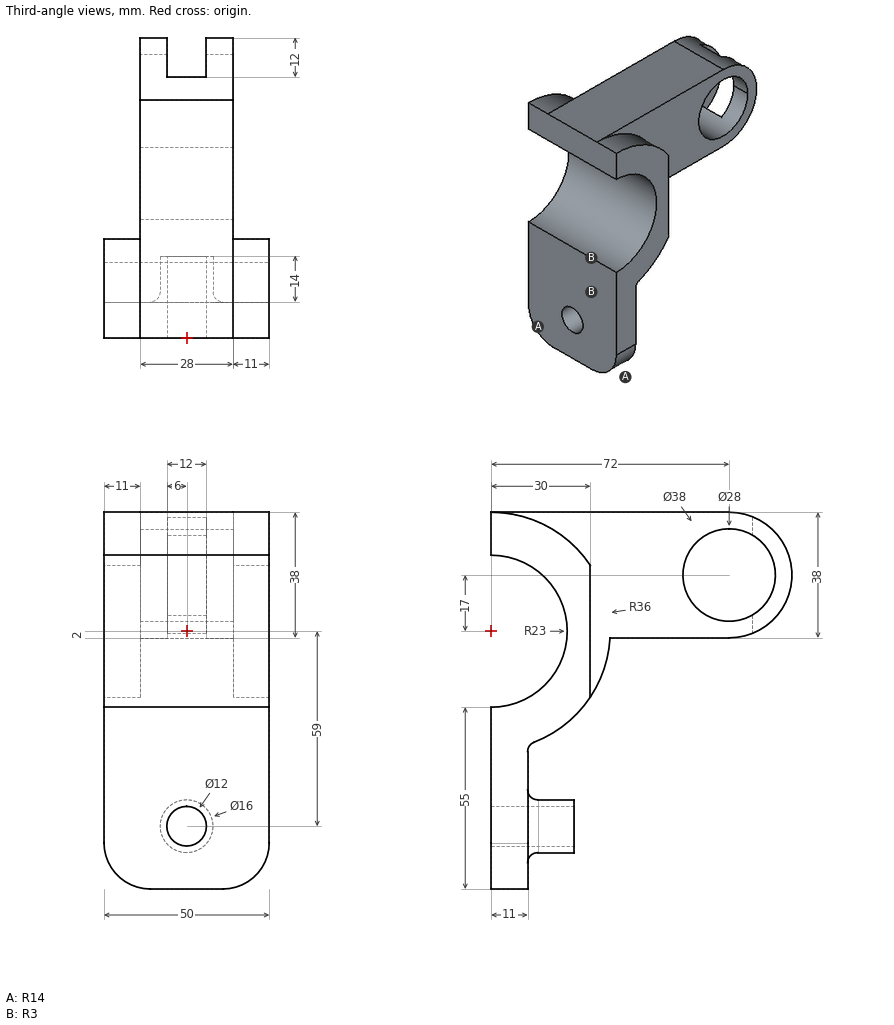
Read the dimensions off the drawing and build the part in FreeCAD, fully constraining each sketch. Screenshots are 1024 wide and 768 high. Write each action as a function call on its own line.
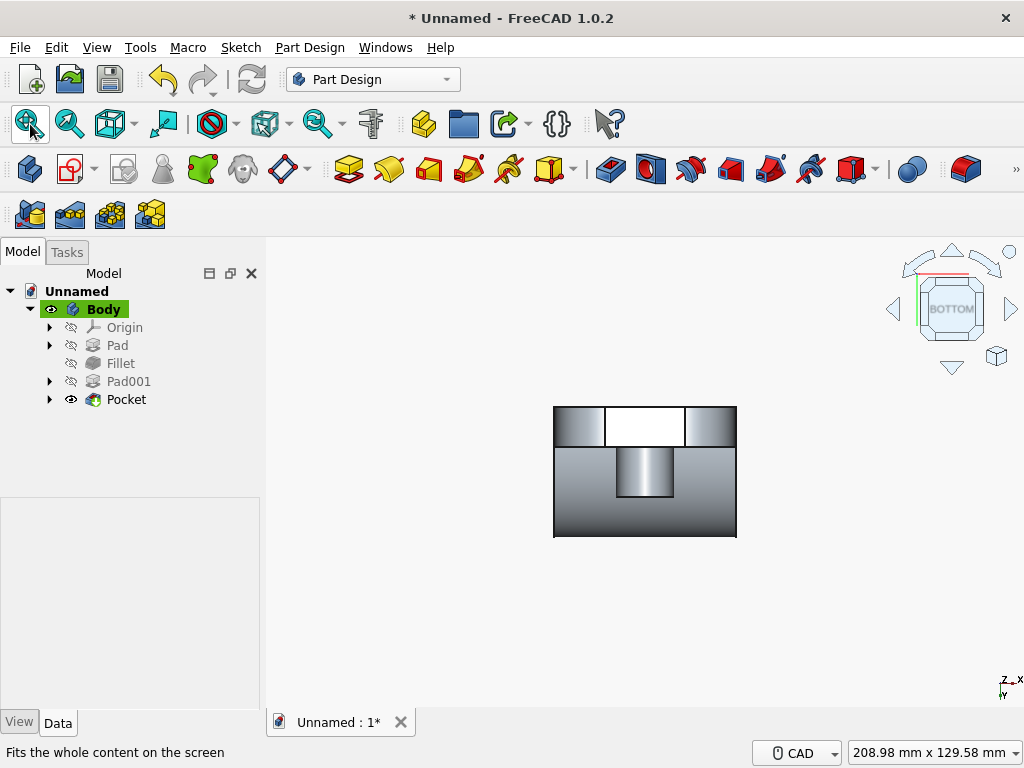
key(4)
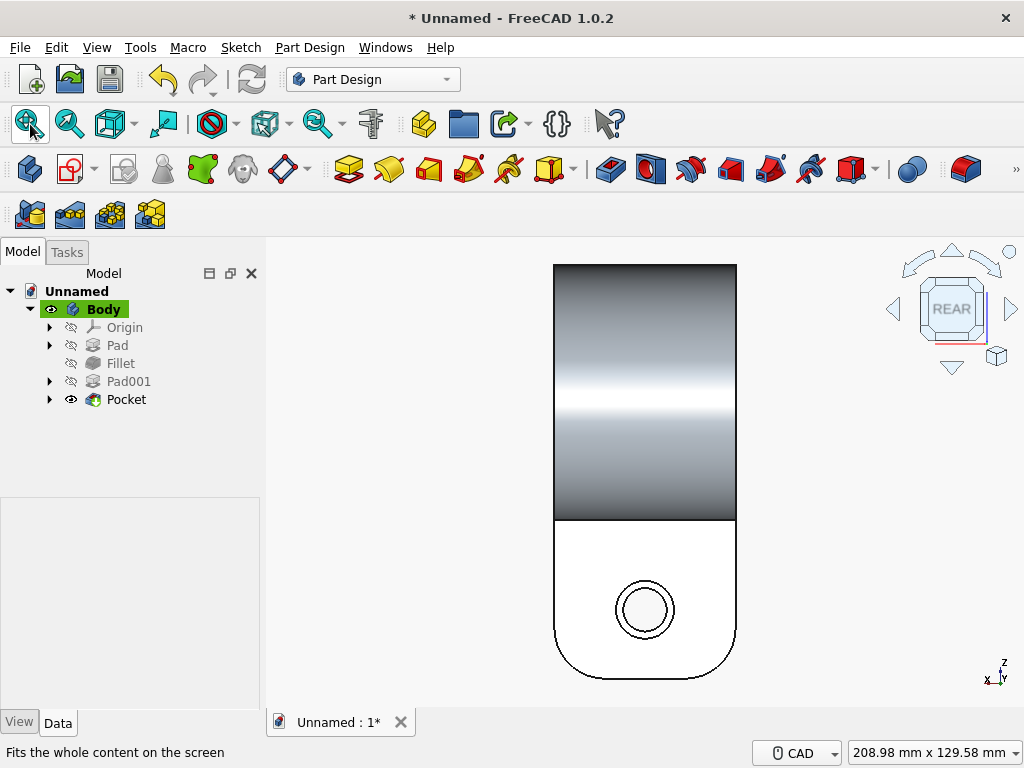
key(6)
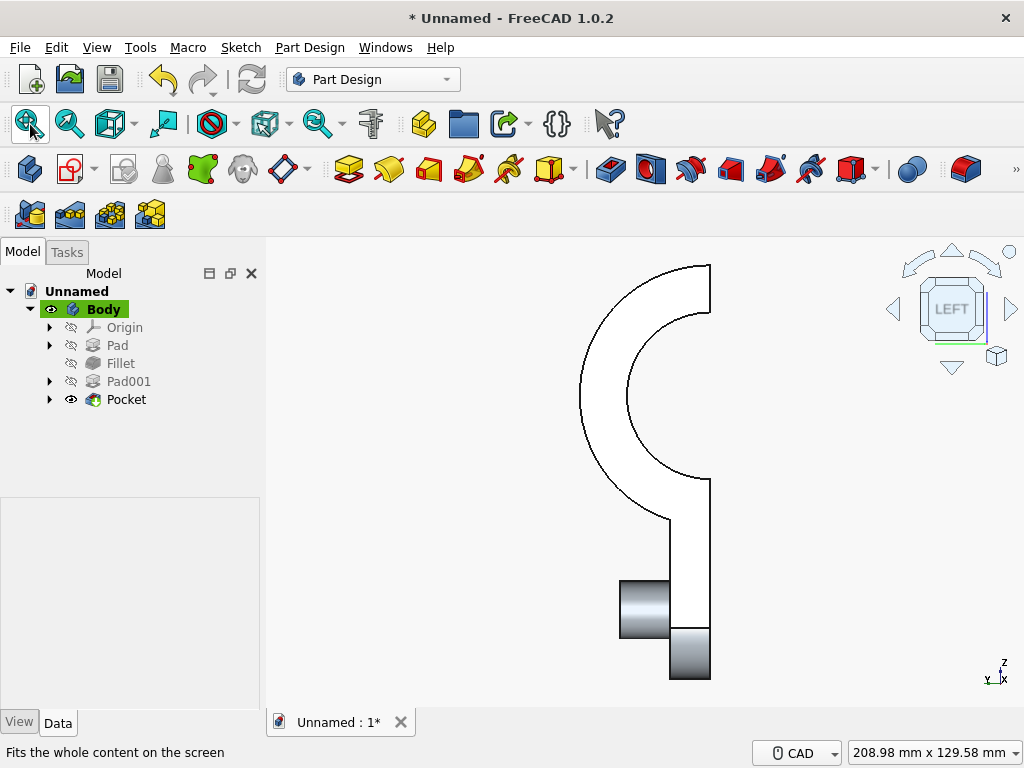
key(v)
key(3)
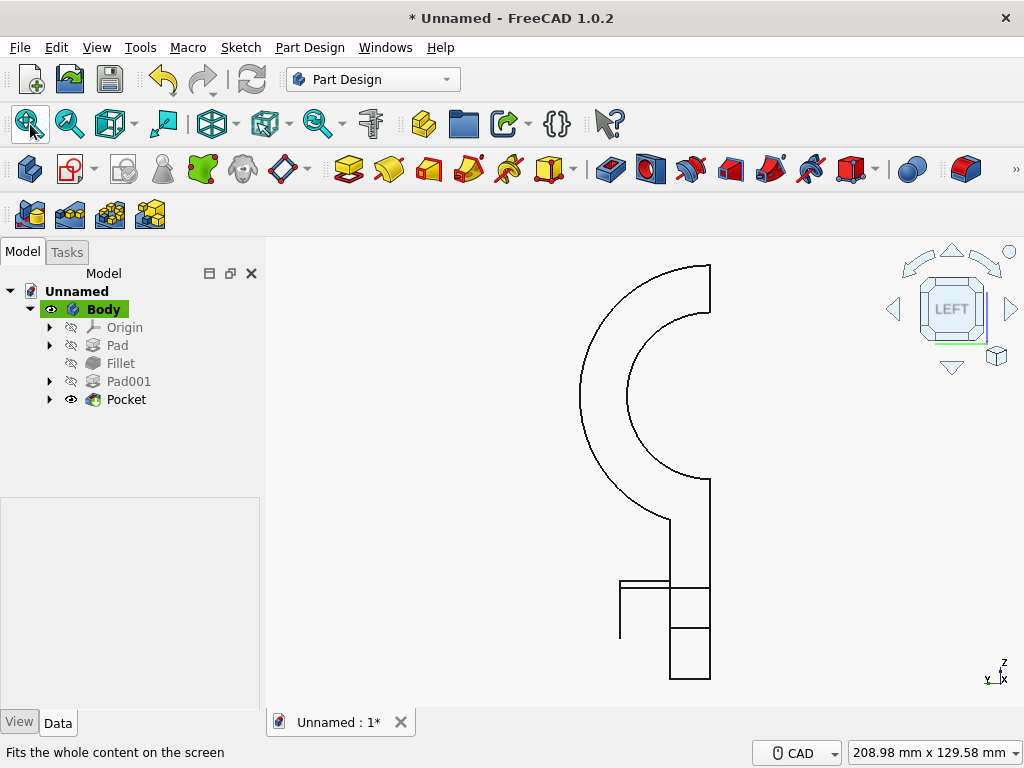
key(0)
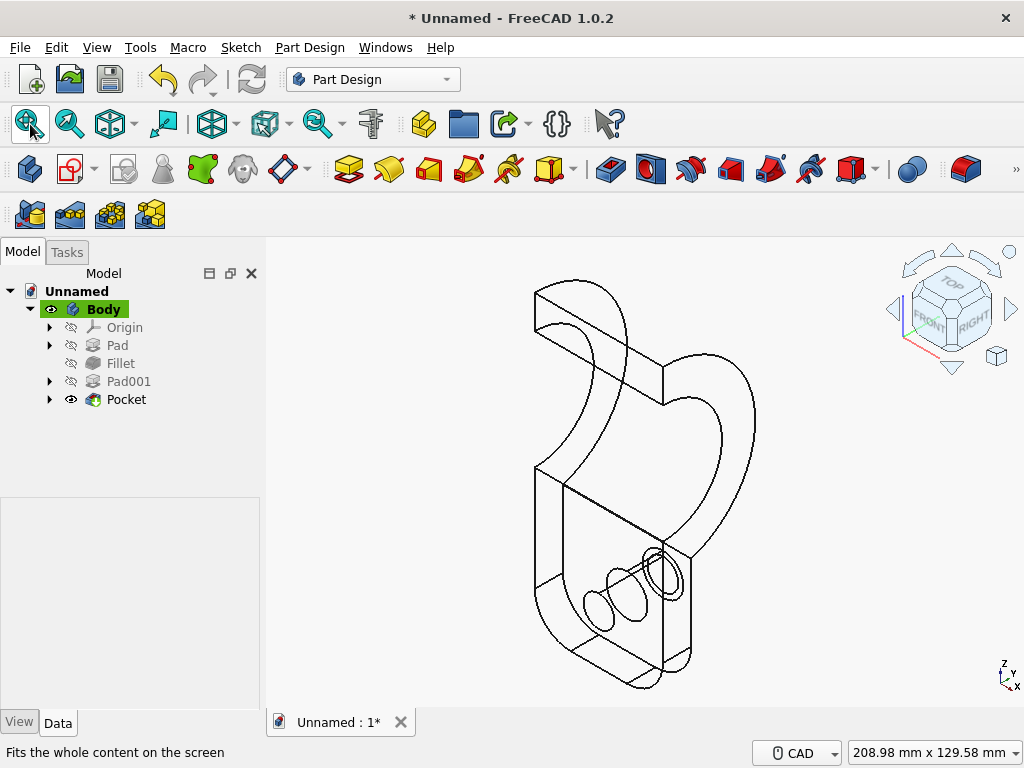
click(676, 549)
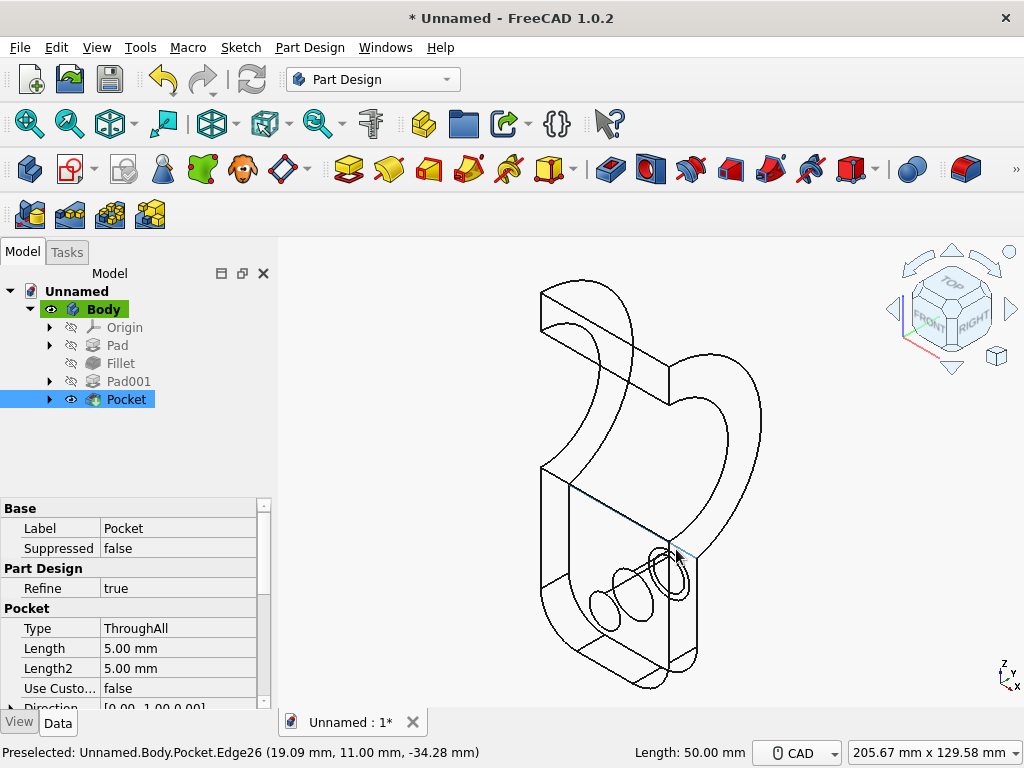
click(633, 618, ctrl)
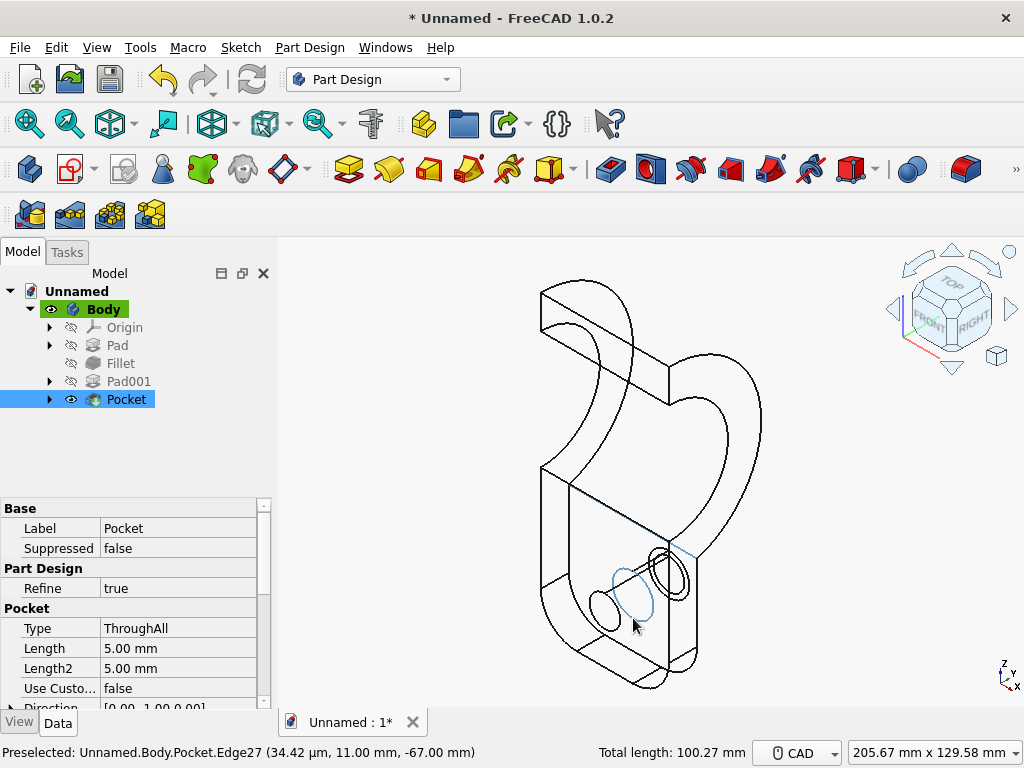
key(v)
key(1)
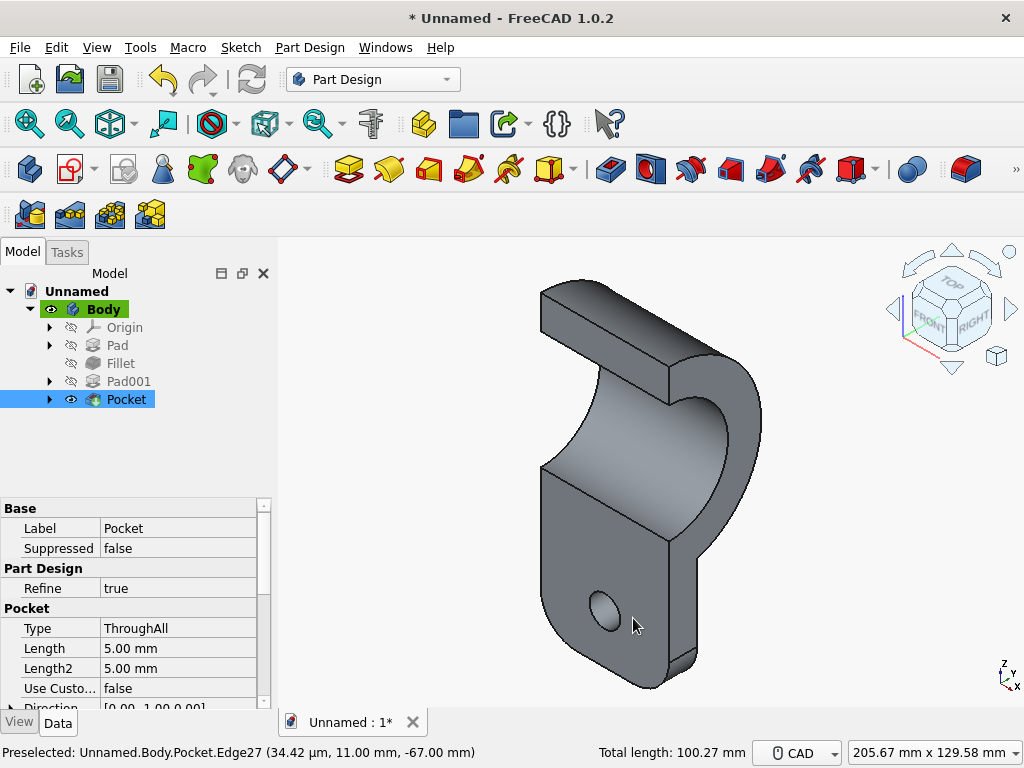
click(966, 170)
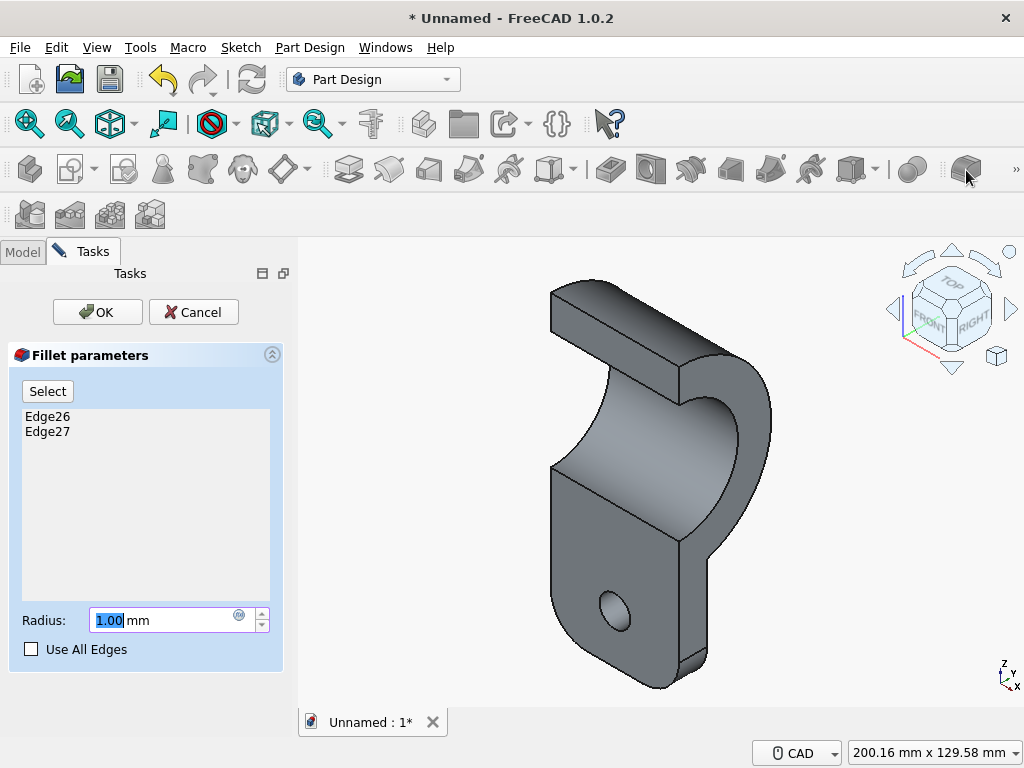
text(3)
key(Tab)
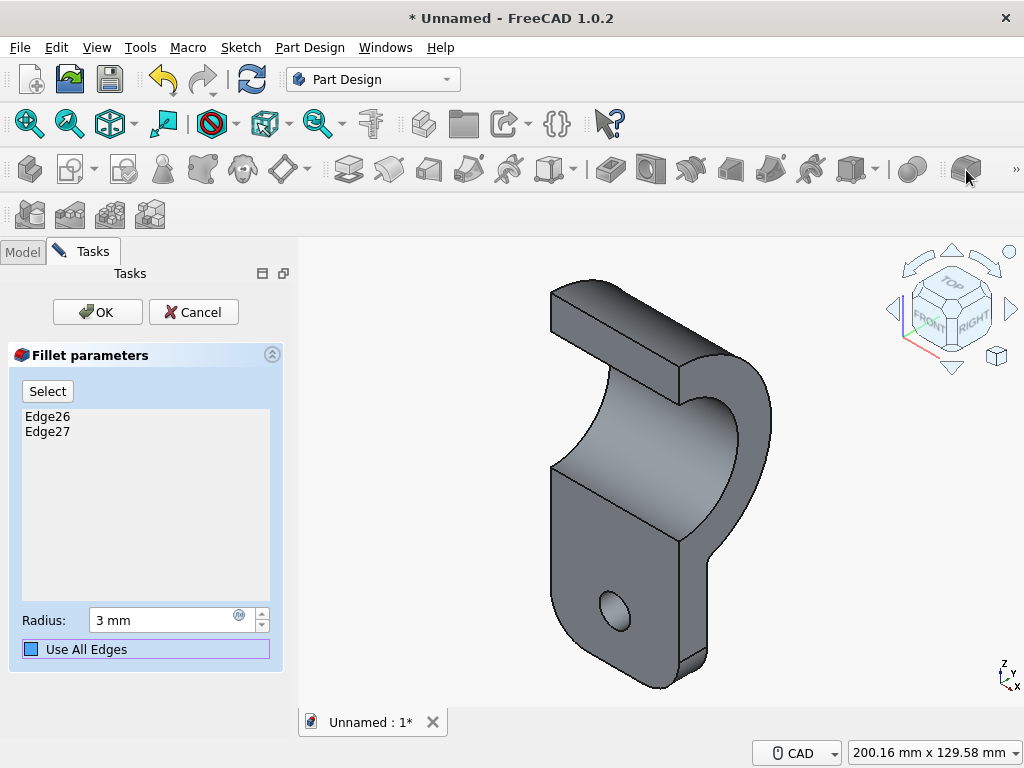
click(98, 312)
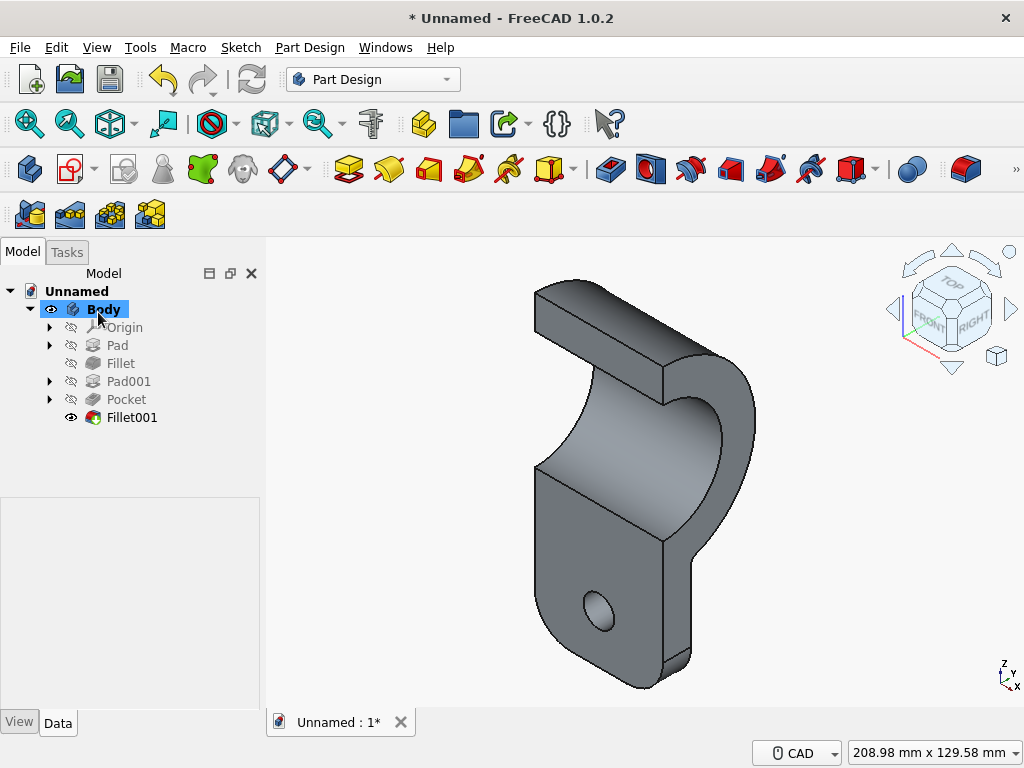
click(70, 170)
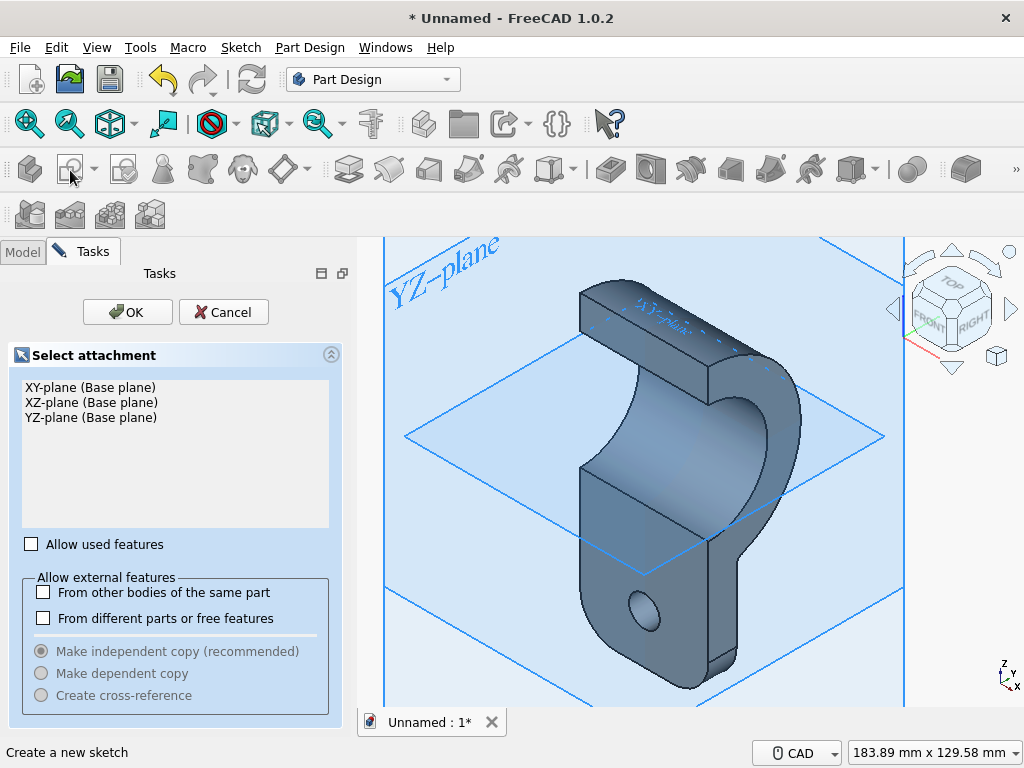
click(82, 418)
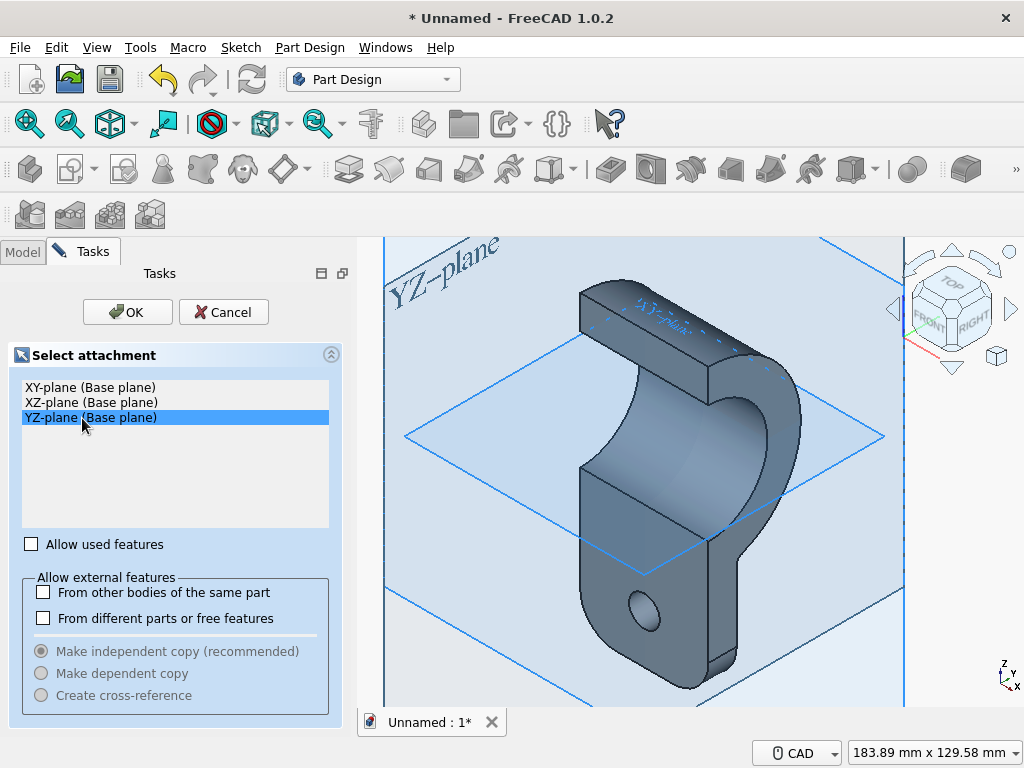
click(128, 312)